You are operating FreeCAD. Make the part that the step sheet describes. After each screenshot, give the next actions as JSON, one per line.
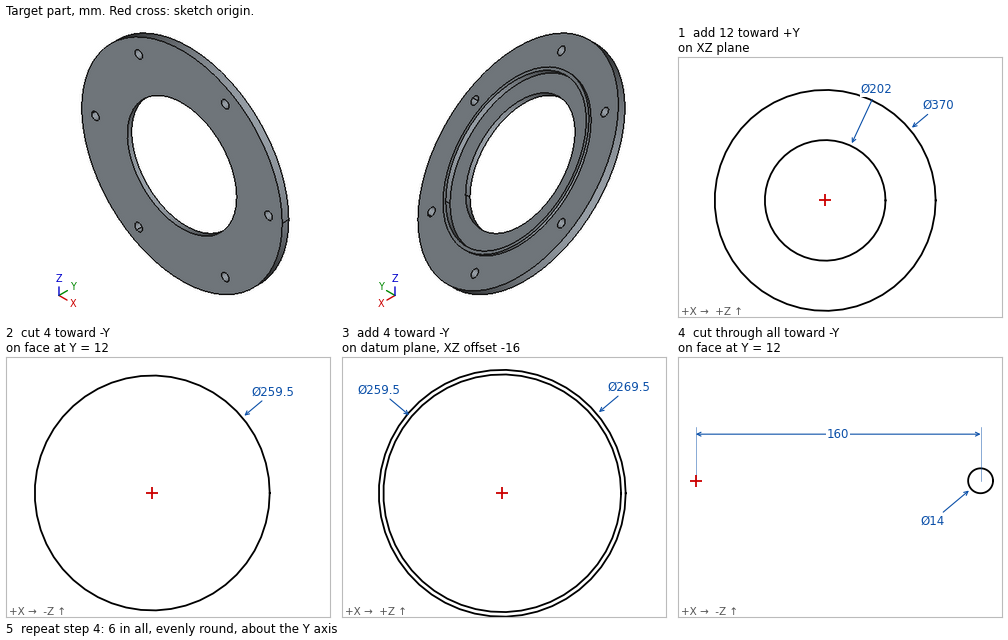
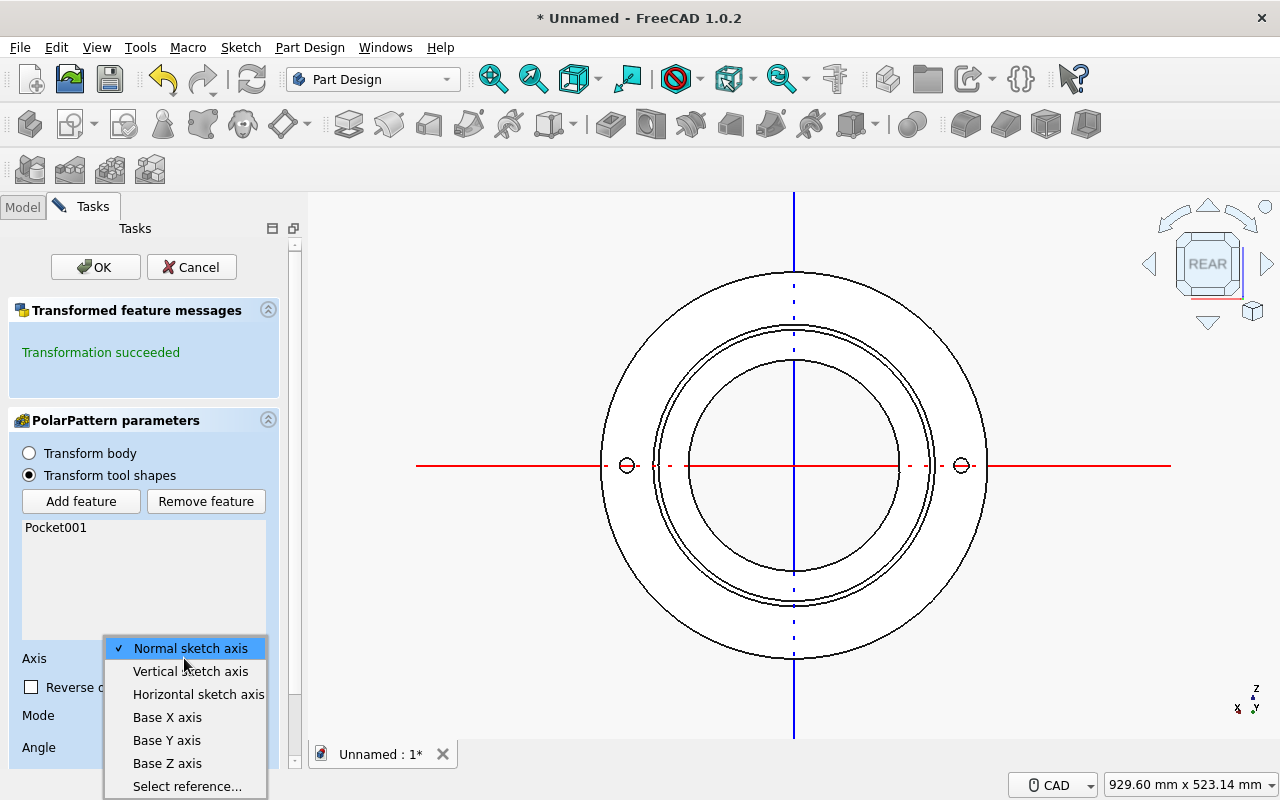
{"action": "left_click", "coordinate": [184, 740]}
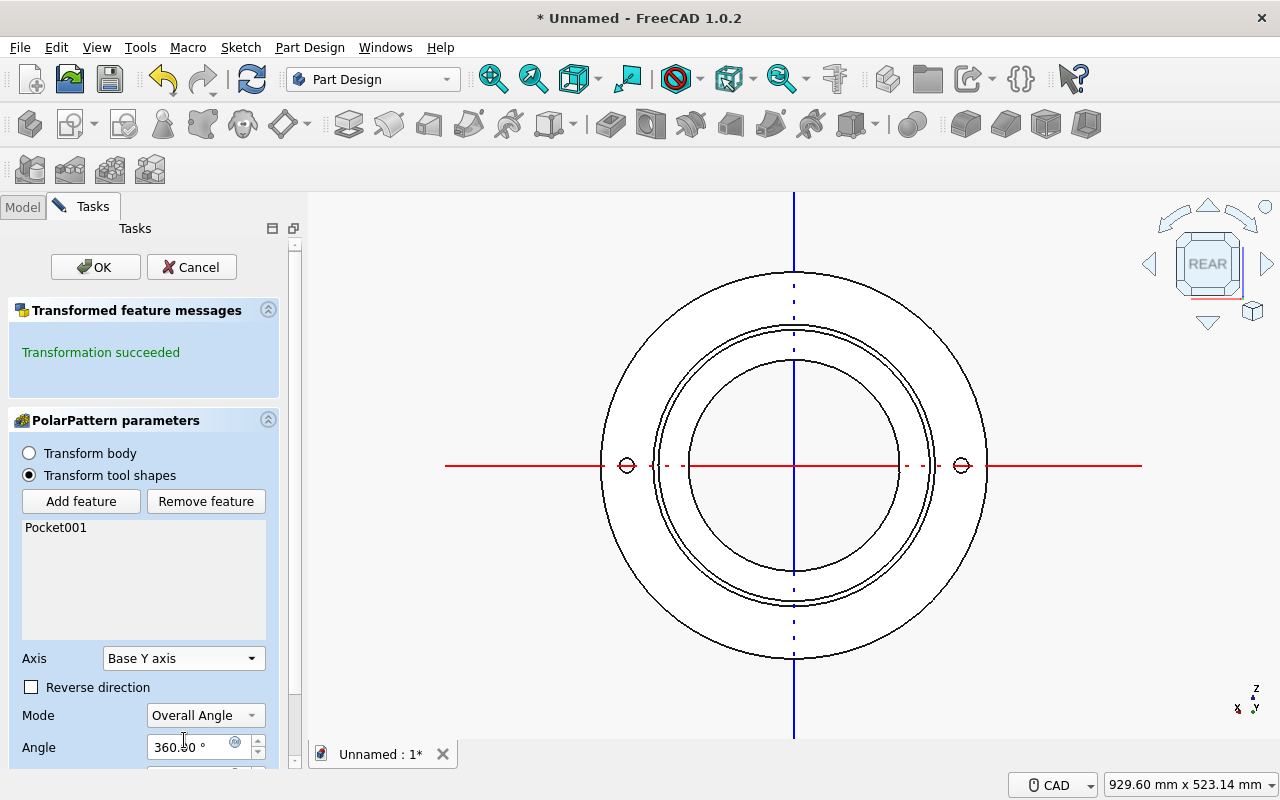
{"action": "scroll", "coordinate": [295, 503], "scroll_direction": "down", "scroll_amount": 2}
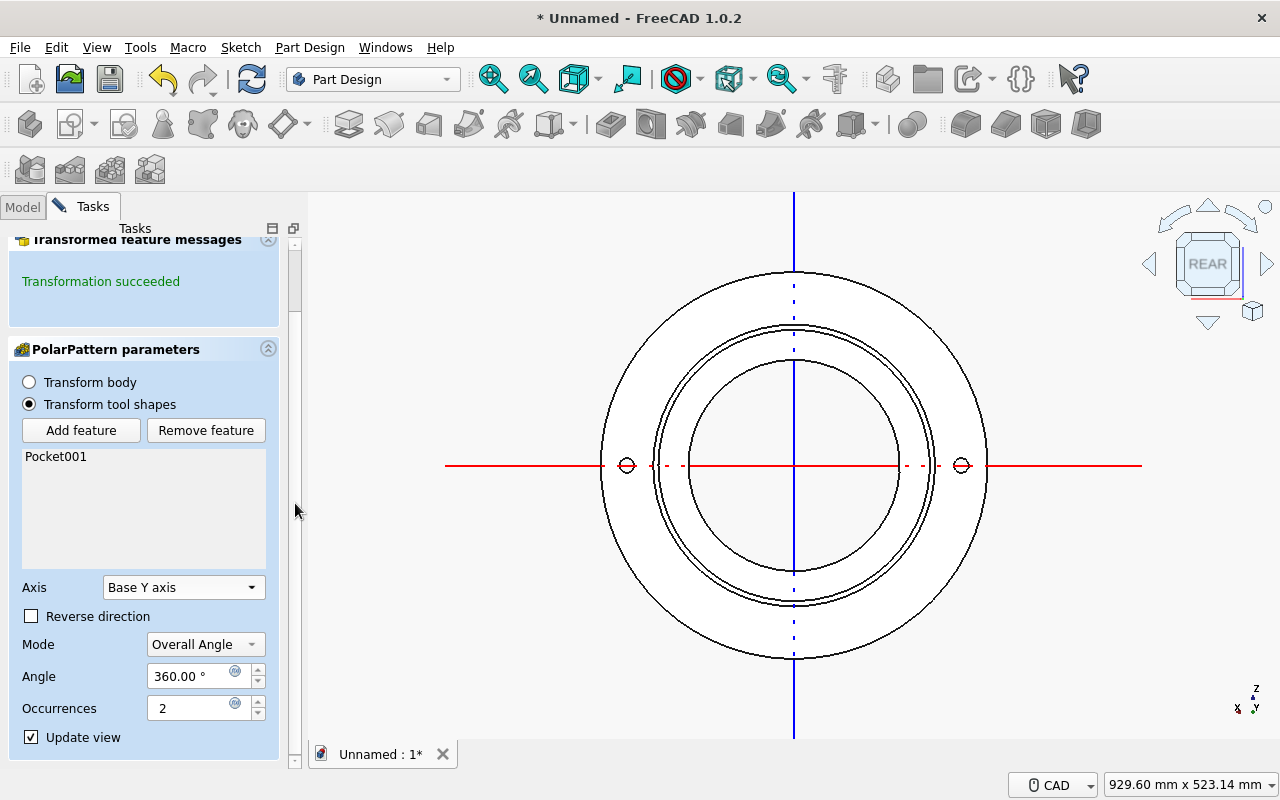
{"action": "triple_click", "coordinate": [198, 708]}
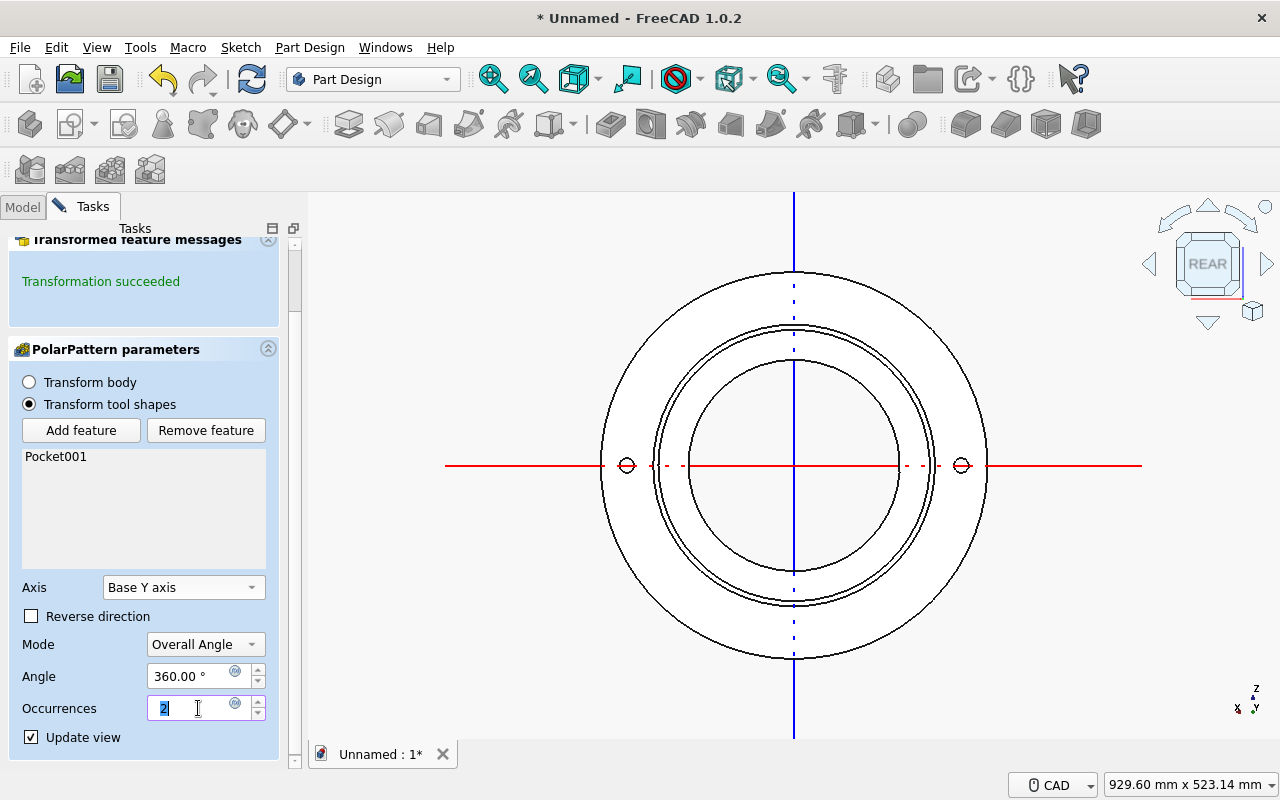
{"action": "type", "text": "6"}
{"action": "key", "text": "Tab"}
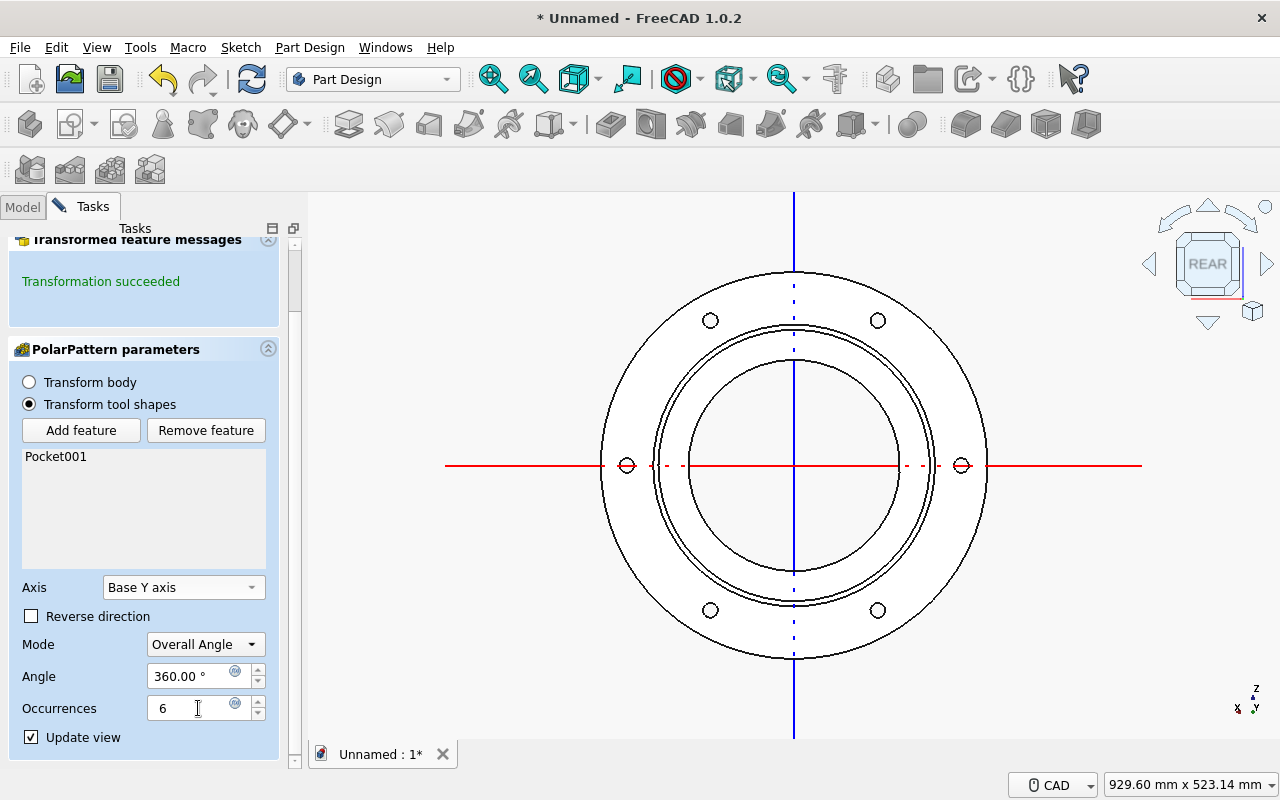
{"action": "scroll", "coordinate": [295, 503], "scroll_direction": "up", "scroll_amount": 2}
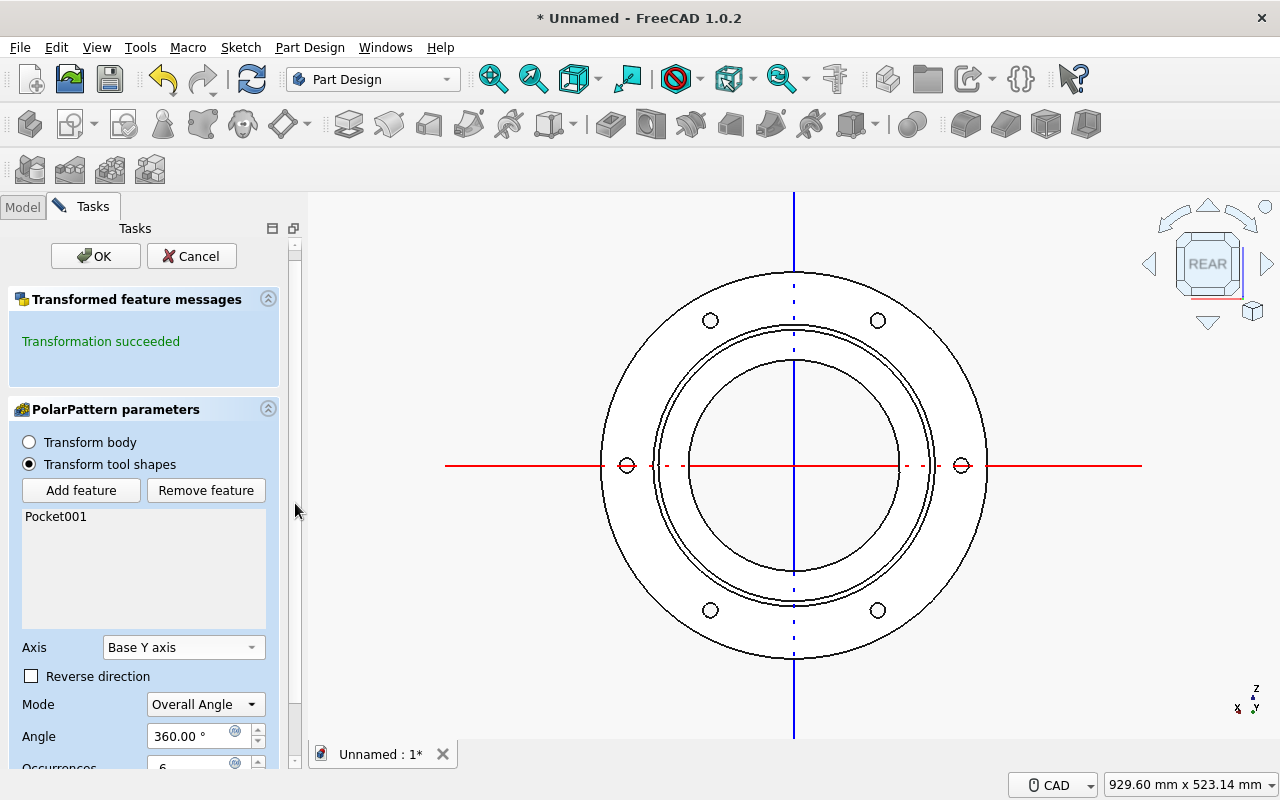
{"action": "left_click", "coordinate": [96, 267]}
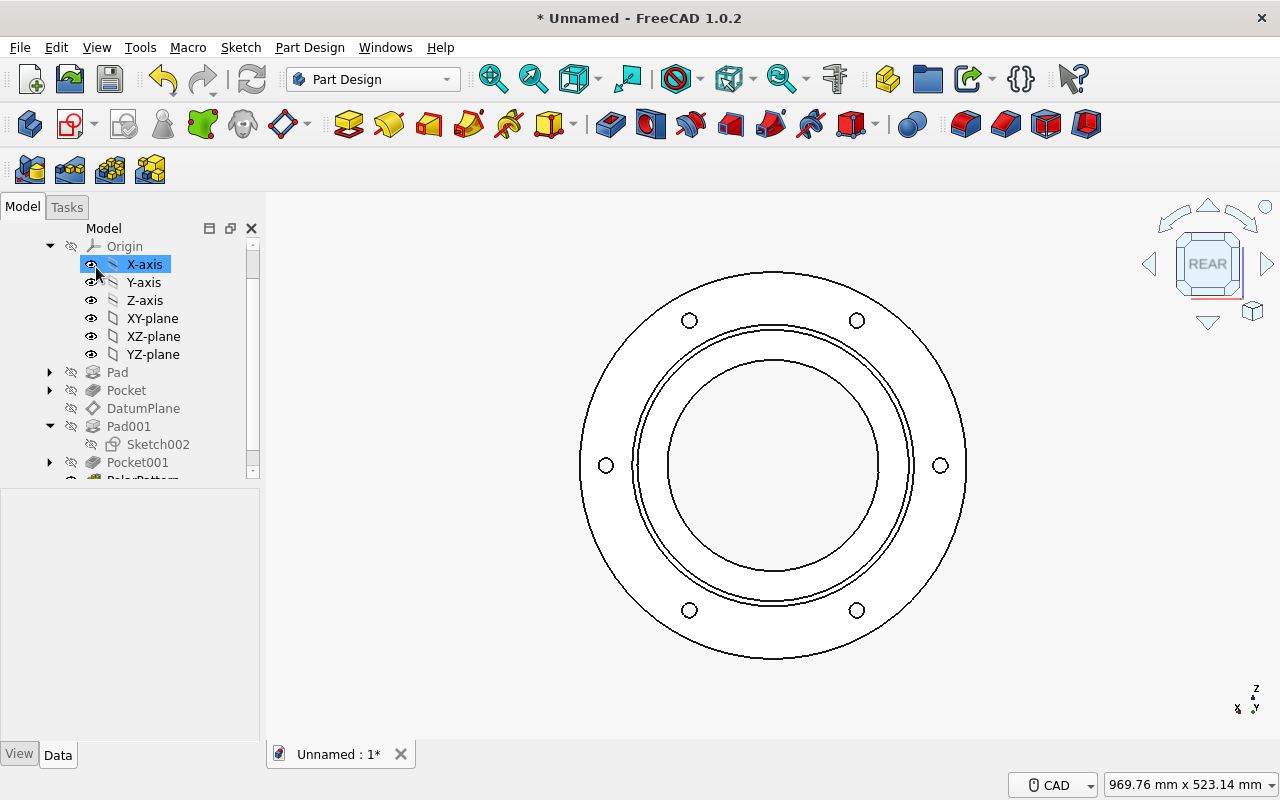
{"action": "key", "text": "0"}